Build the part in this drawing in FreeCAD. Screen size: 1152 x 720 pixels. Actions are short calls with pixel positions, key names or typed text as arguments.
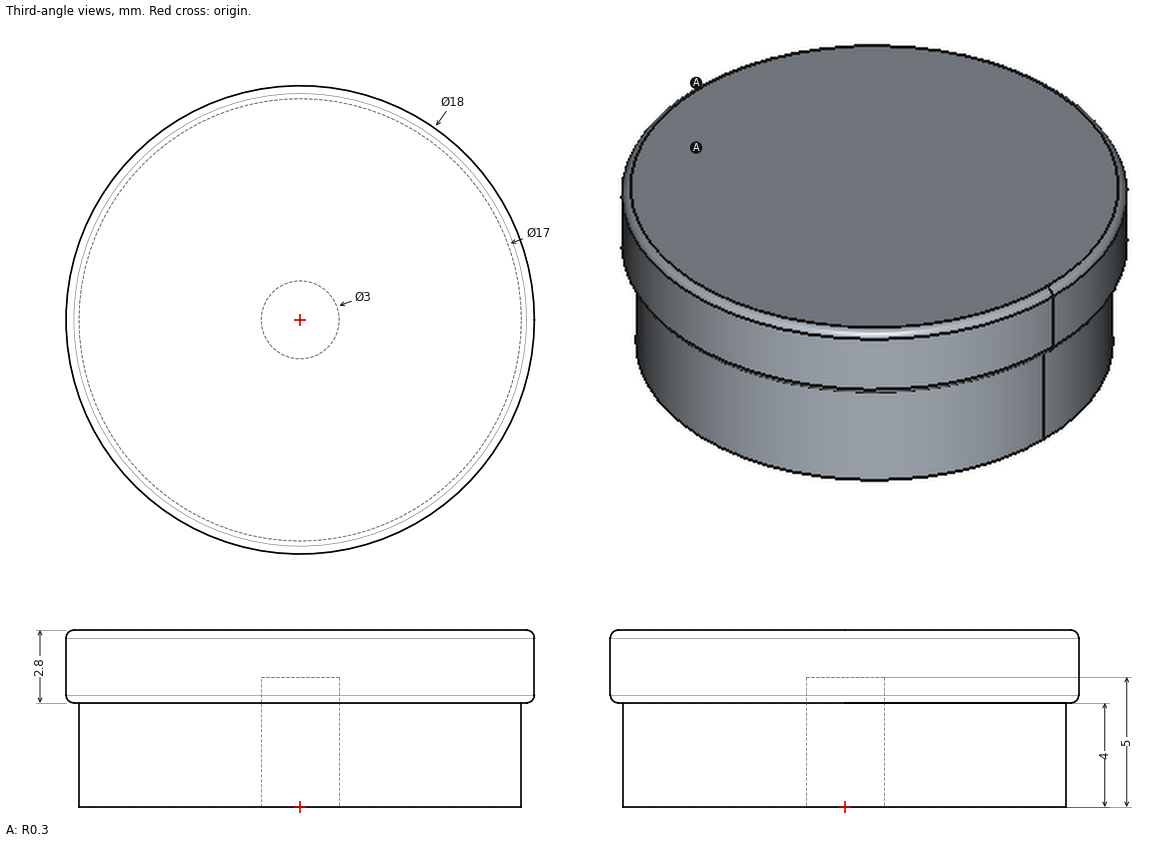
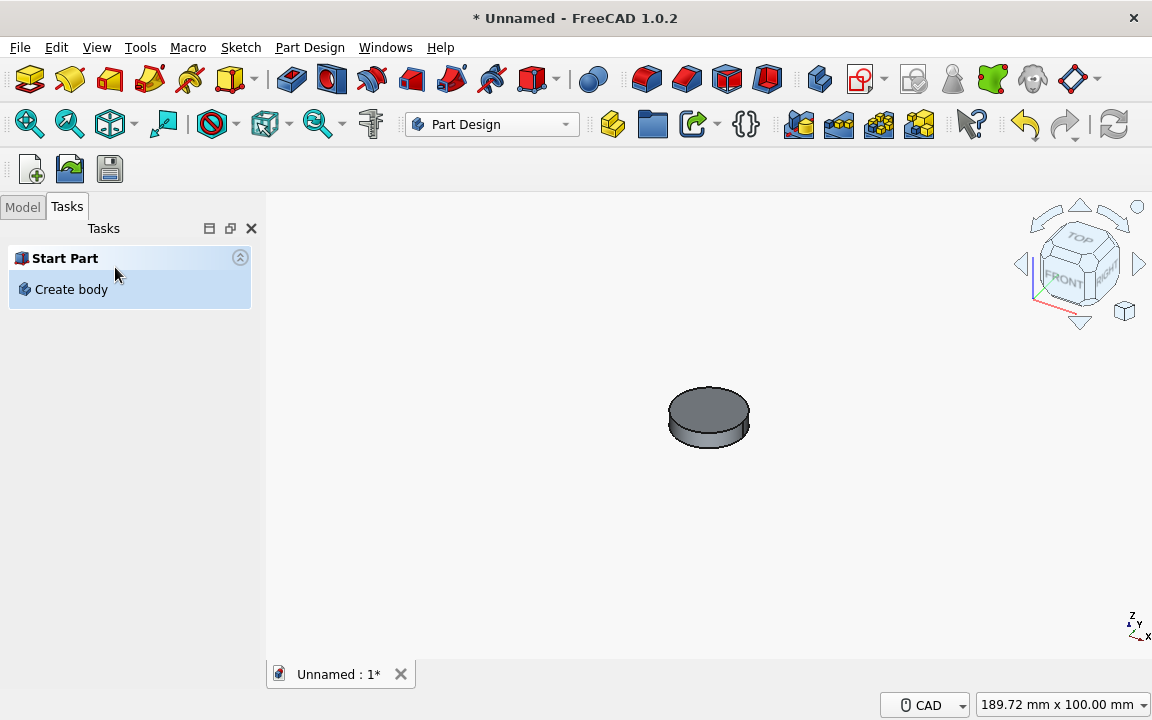
key(v)
key(f)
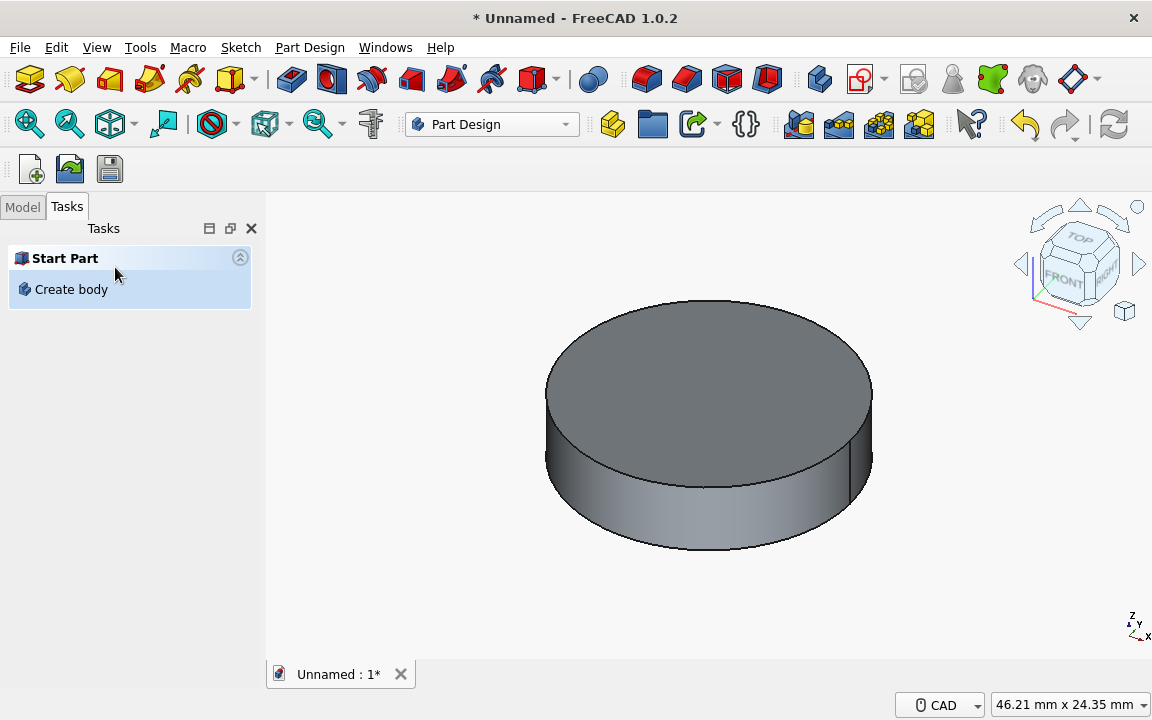
click(709, 393)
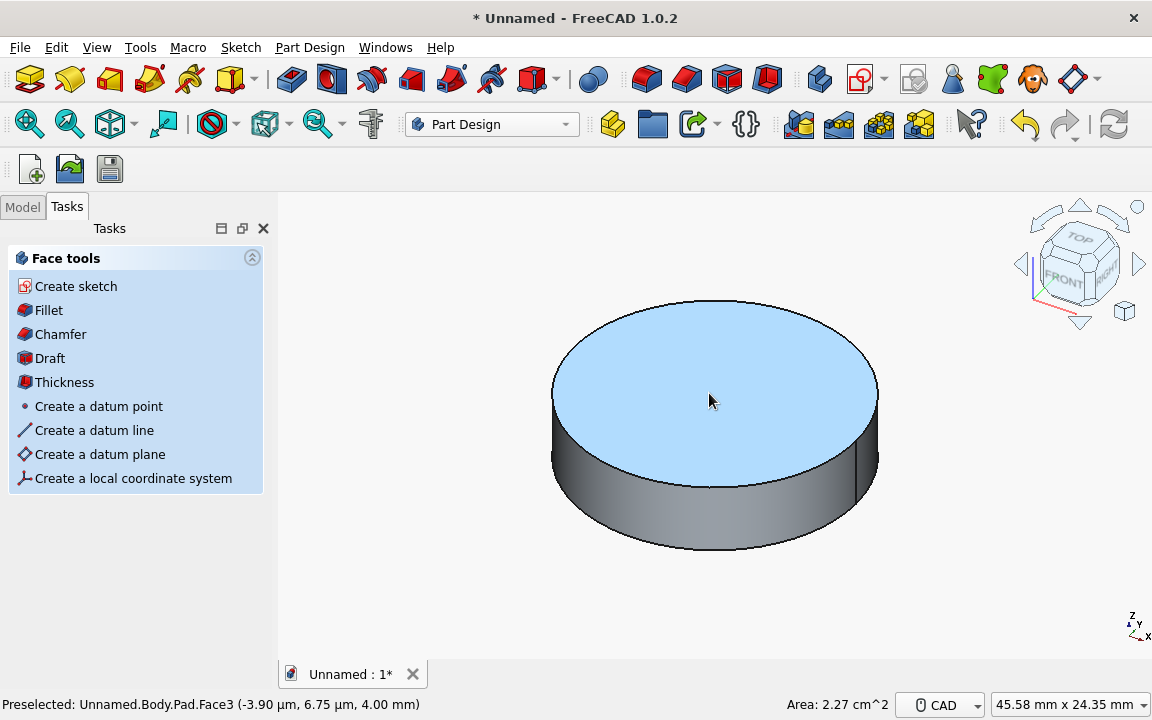
click(860, 80)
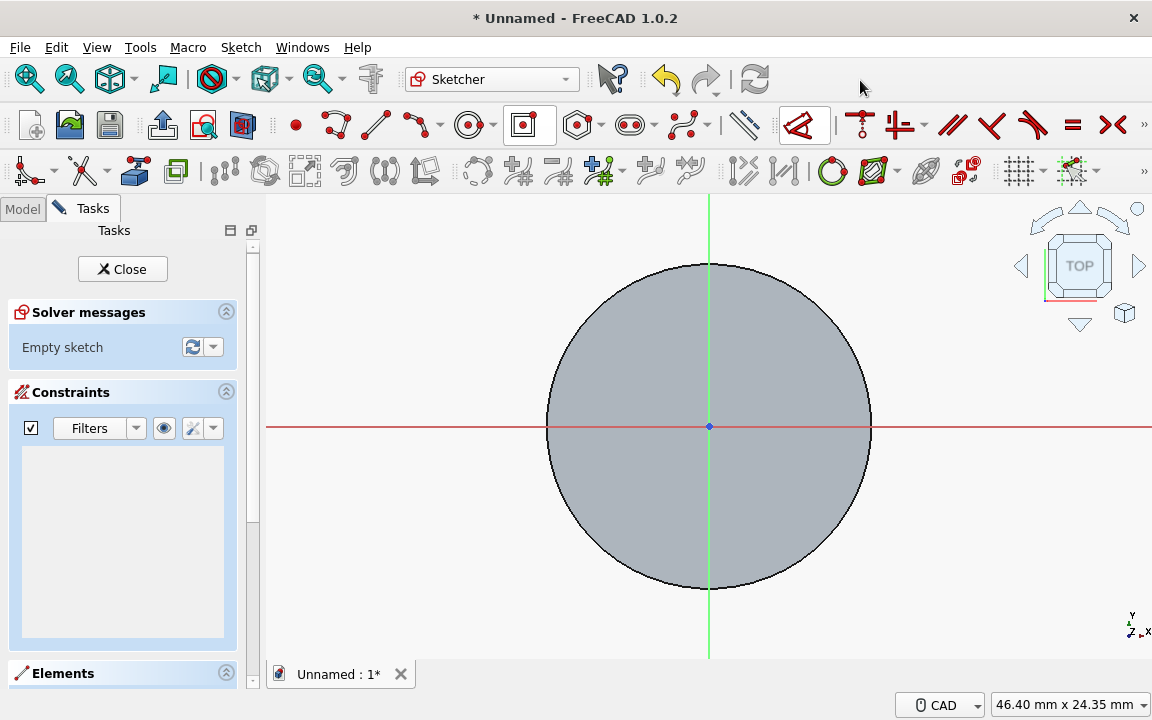
key(g)
key(c)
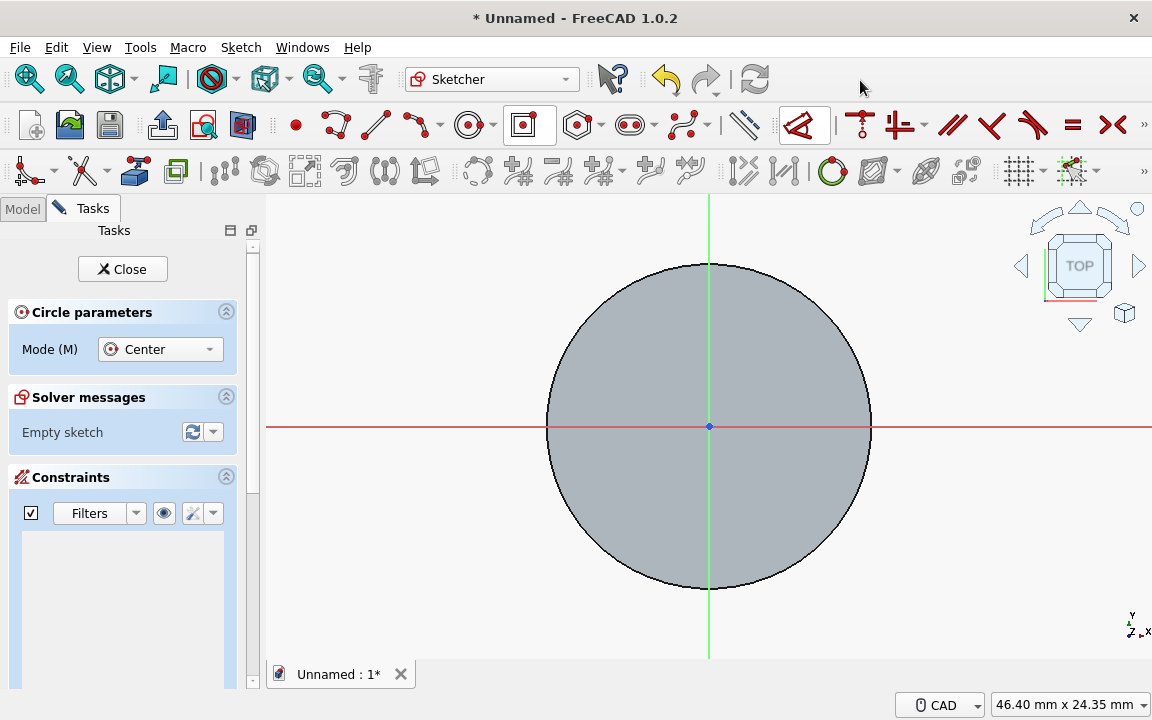
click(709, 426)
move(831, 305)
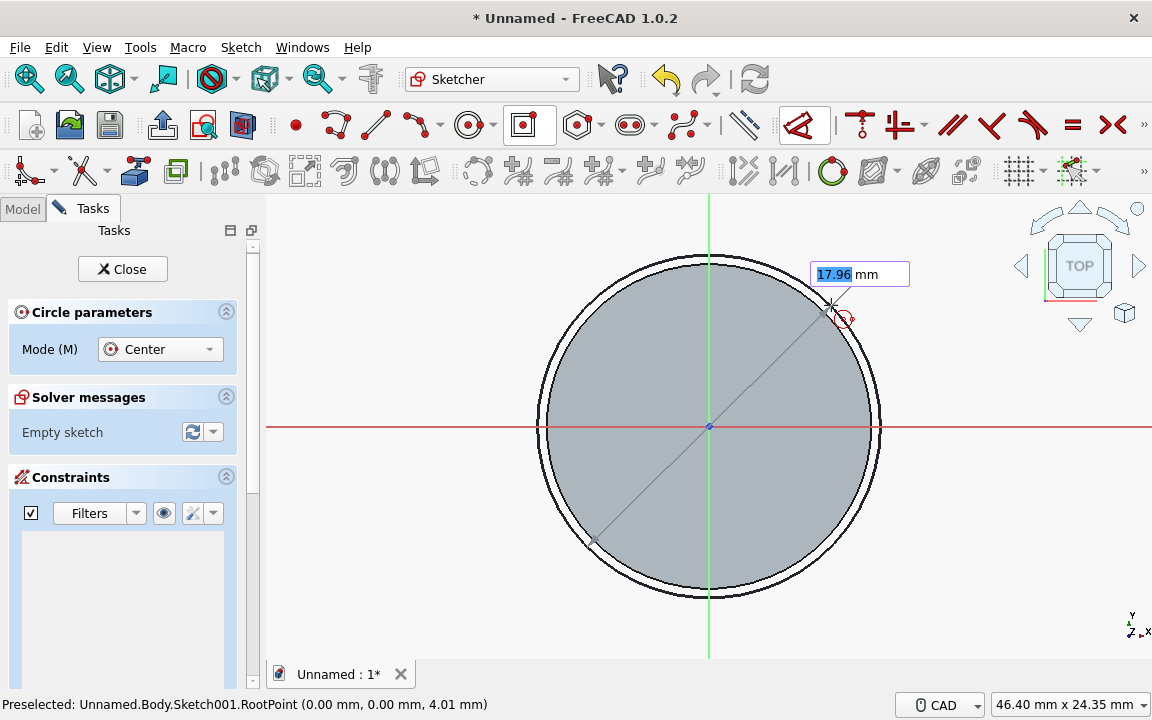
text(18)
key(Return)
key(Escape)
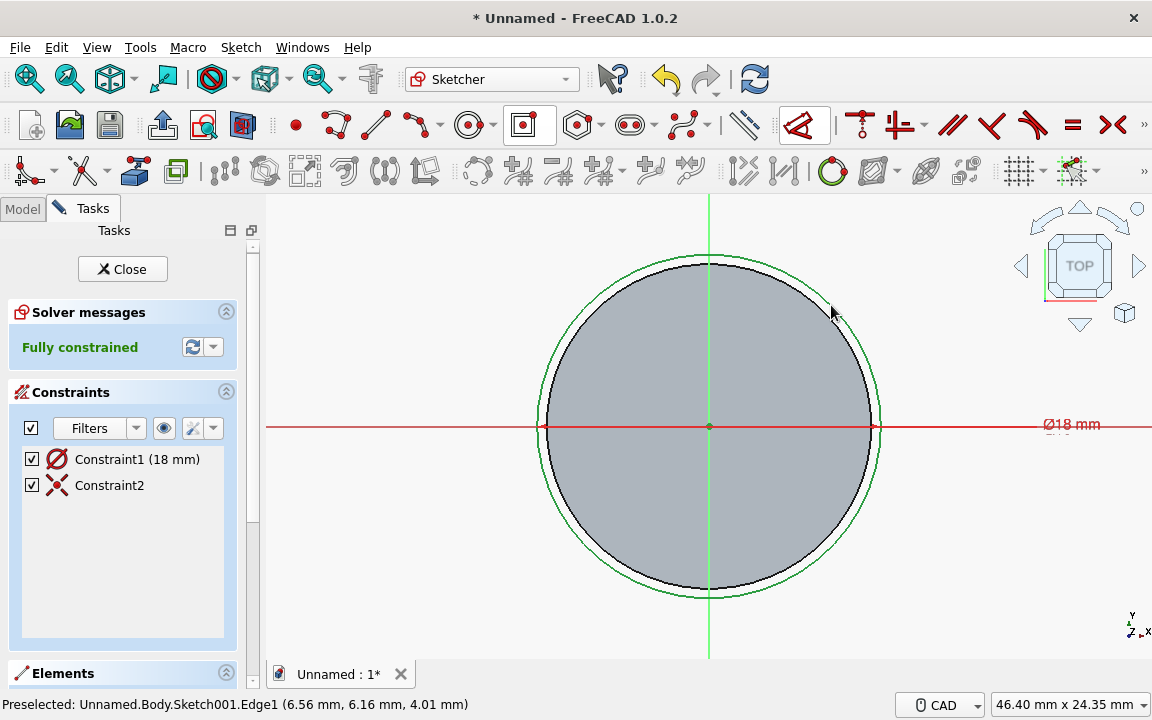
click(123, 269)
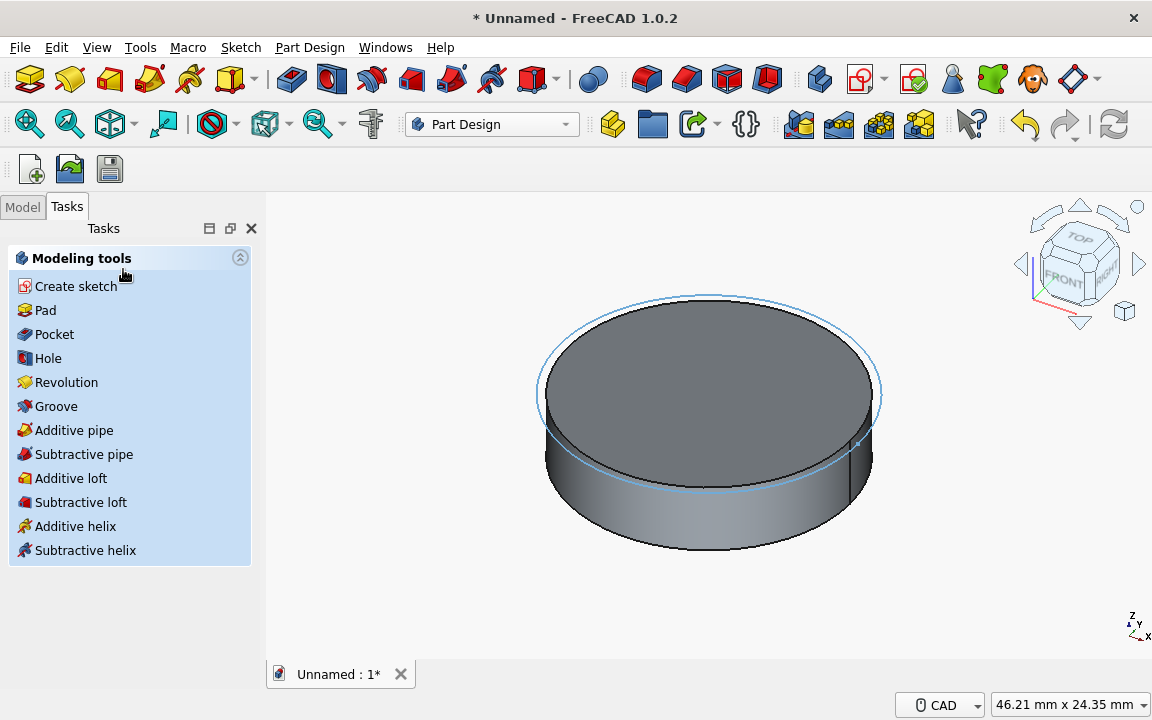
click(30, 80)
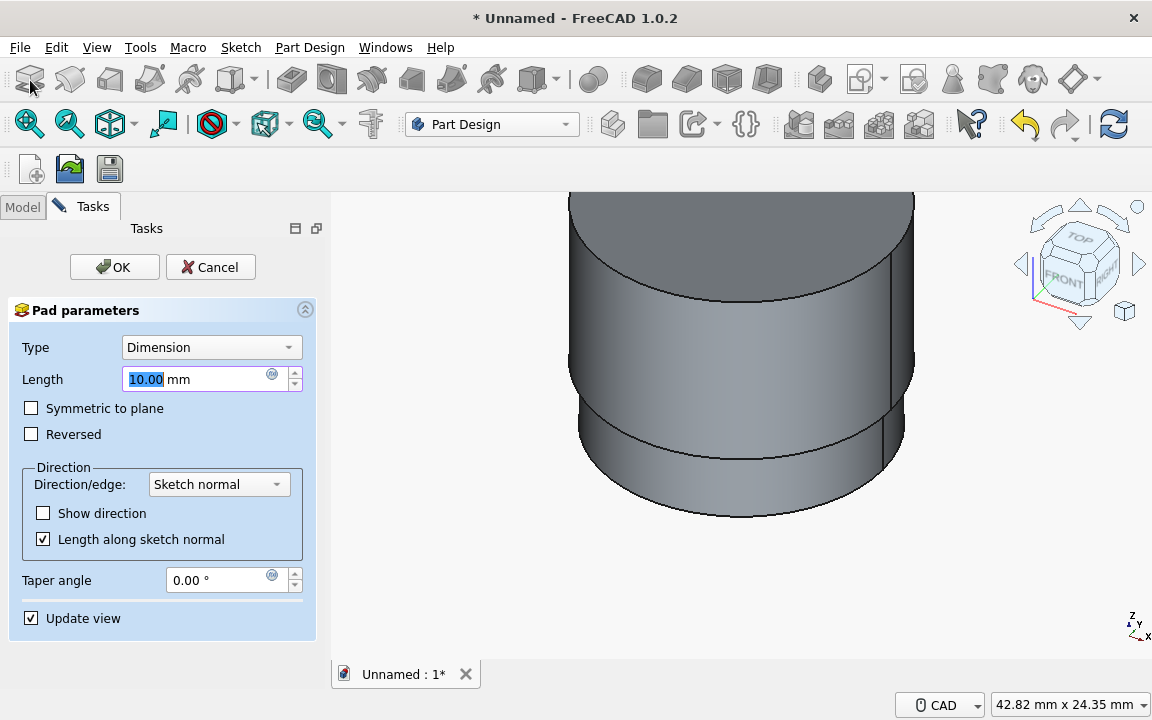
text(2.8)
key(Tab)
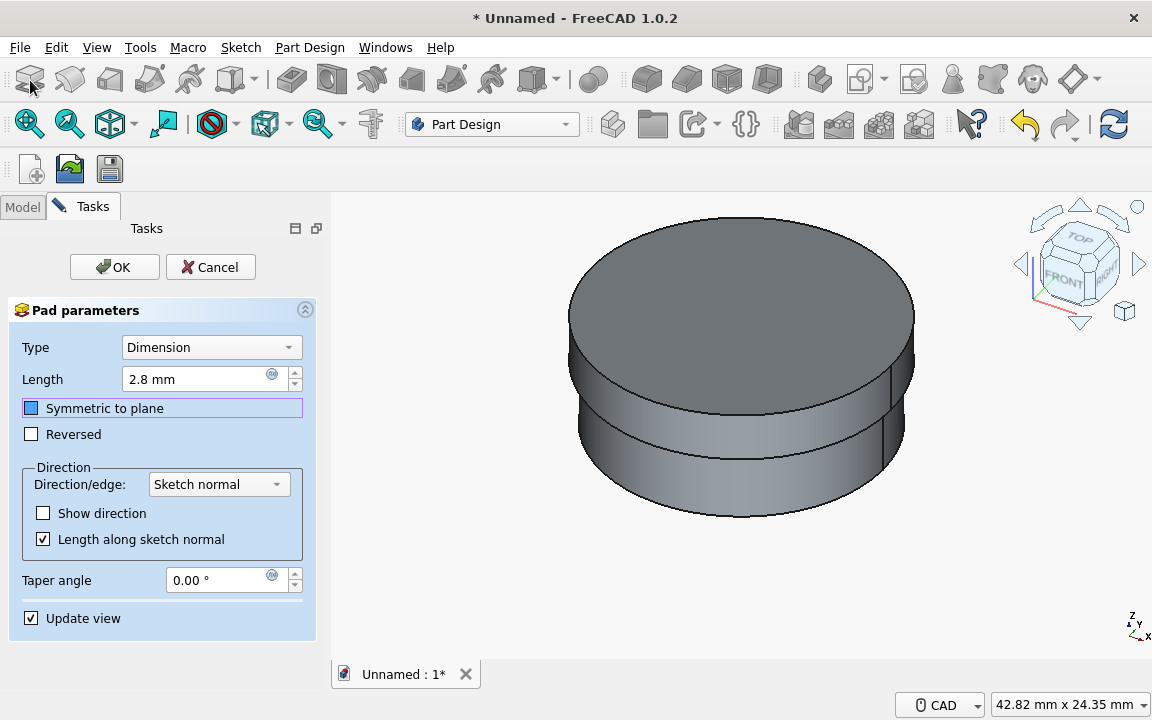
click(115, 267)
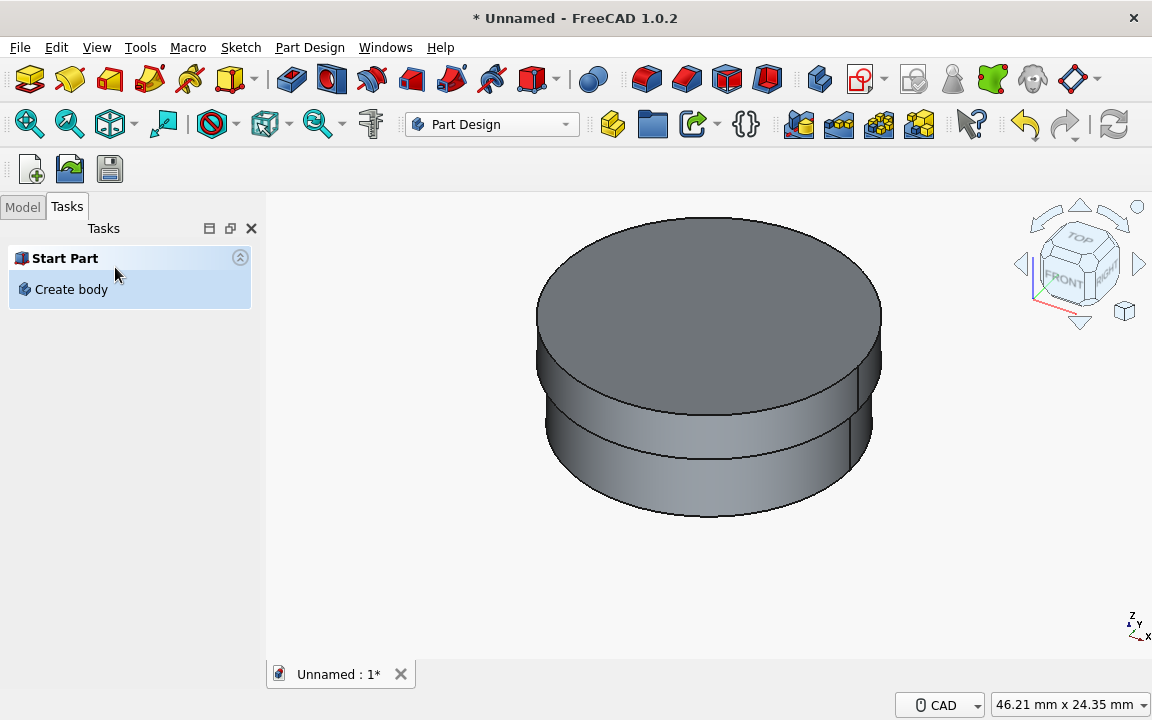
key(v)
key(f)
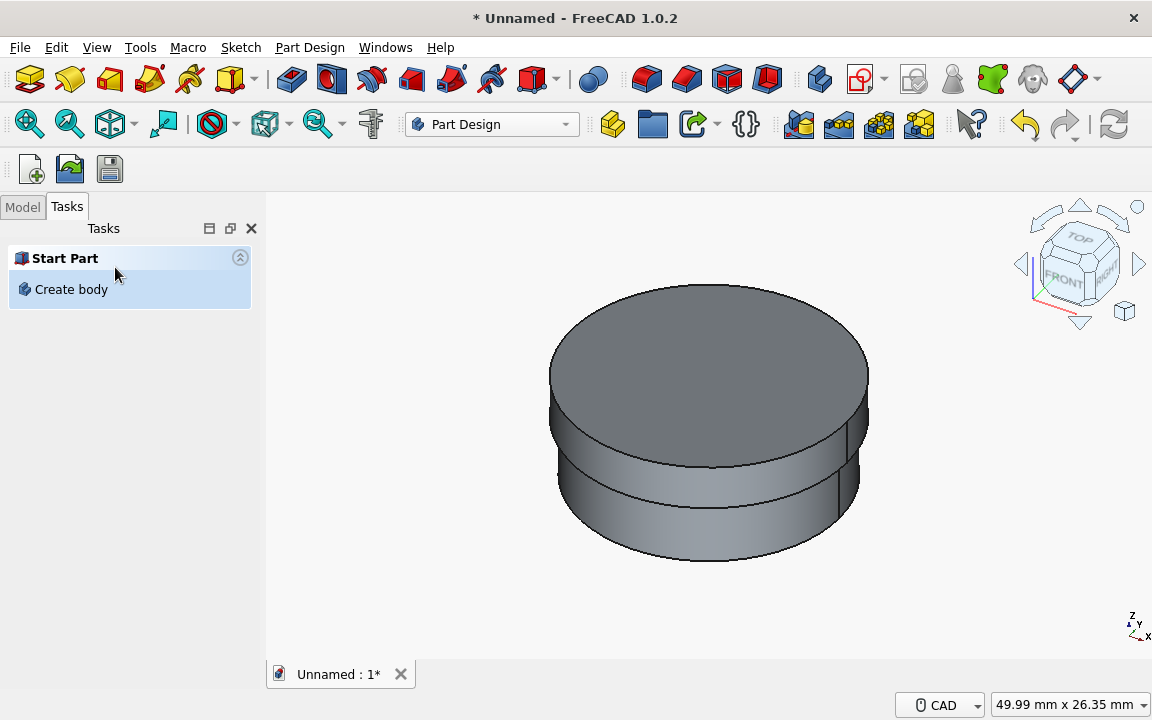
click(550, 385)